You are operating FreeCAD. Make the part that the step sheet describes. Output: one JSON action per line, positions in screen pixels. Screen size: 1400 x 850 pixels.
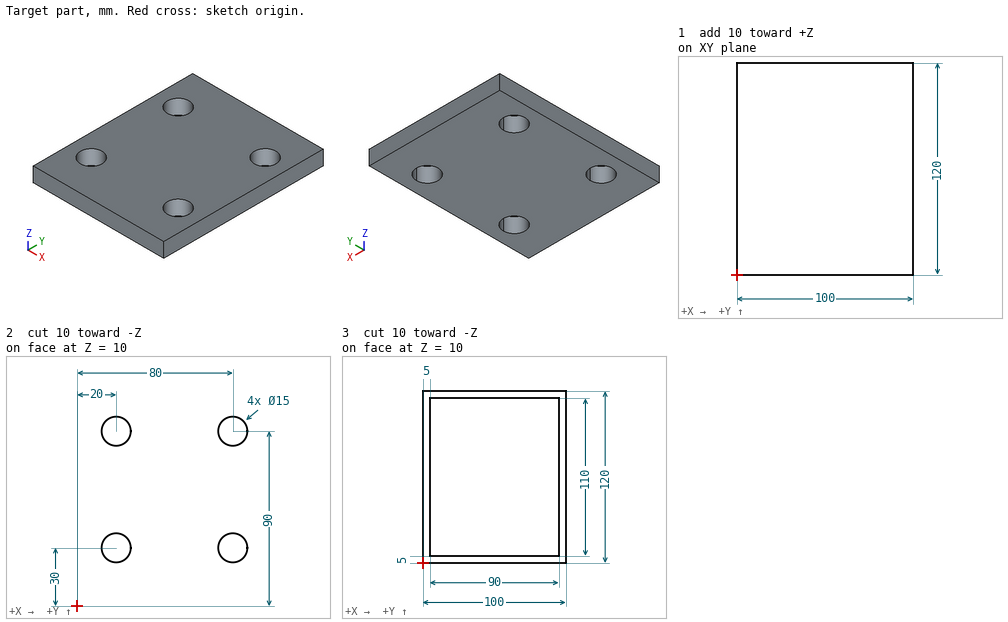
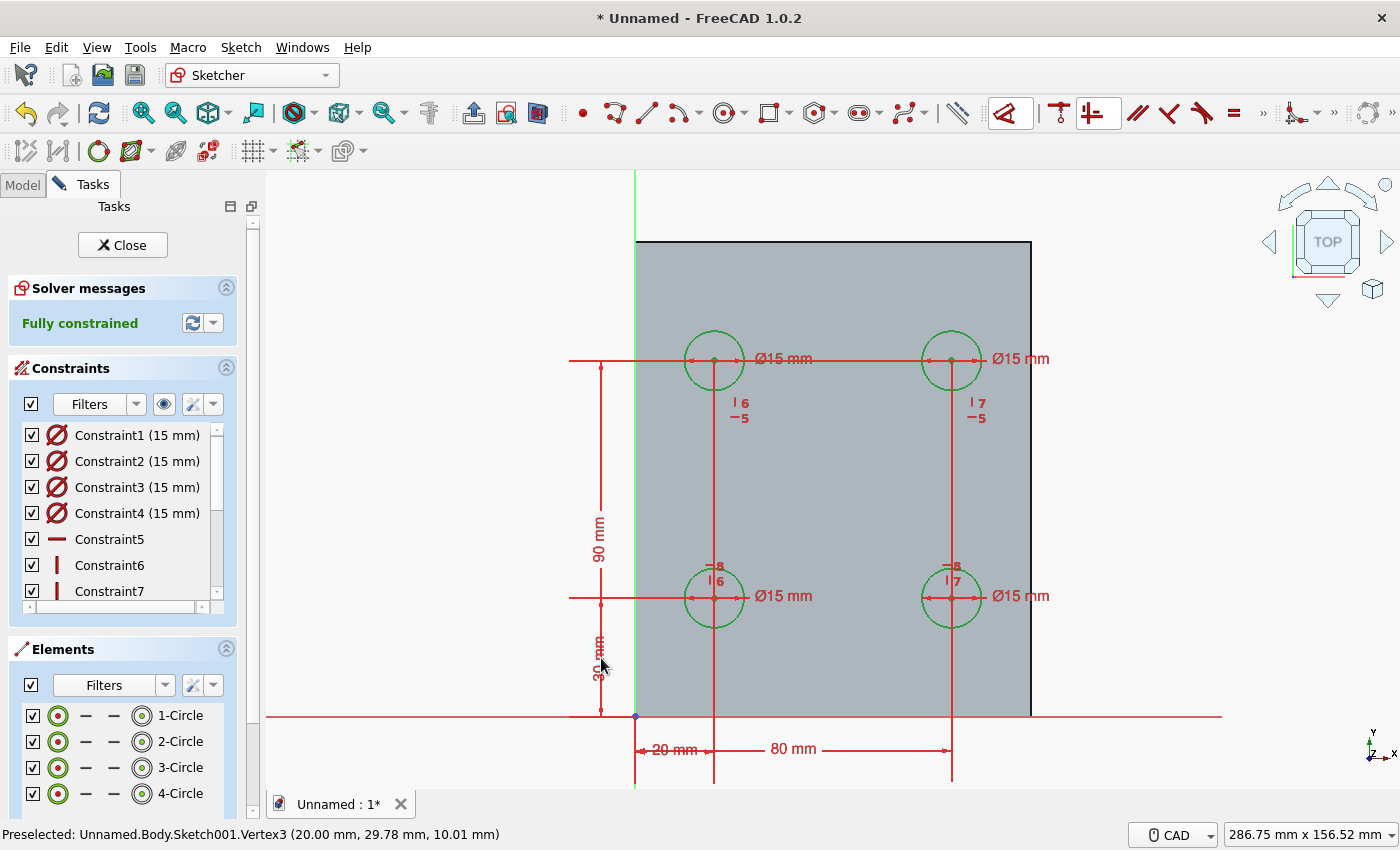
{"action": "left_click", "coordinate": [123, 245]}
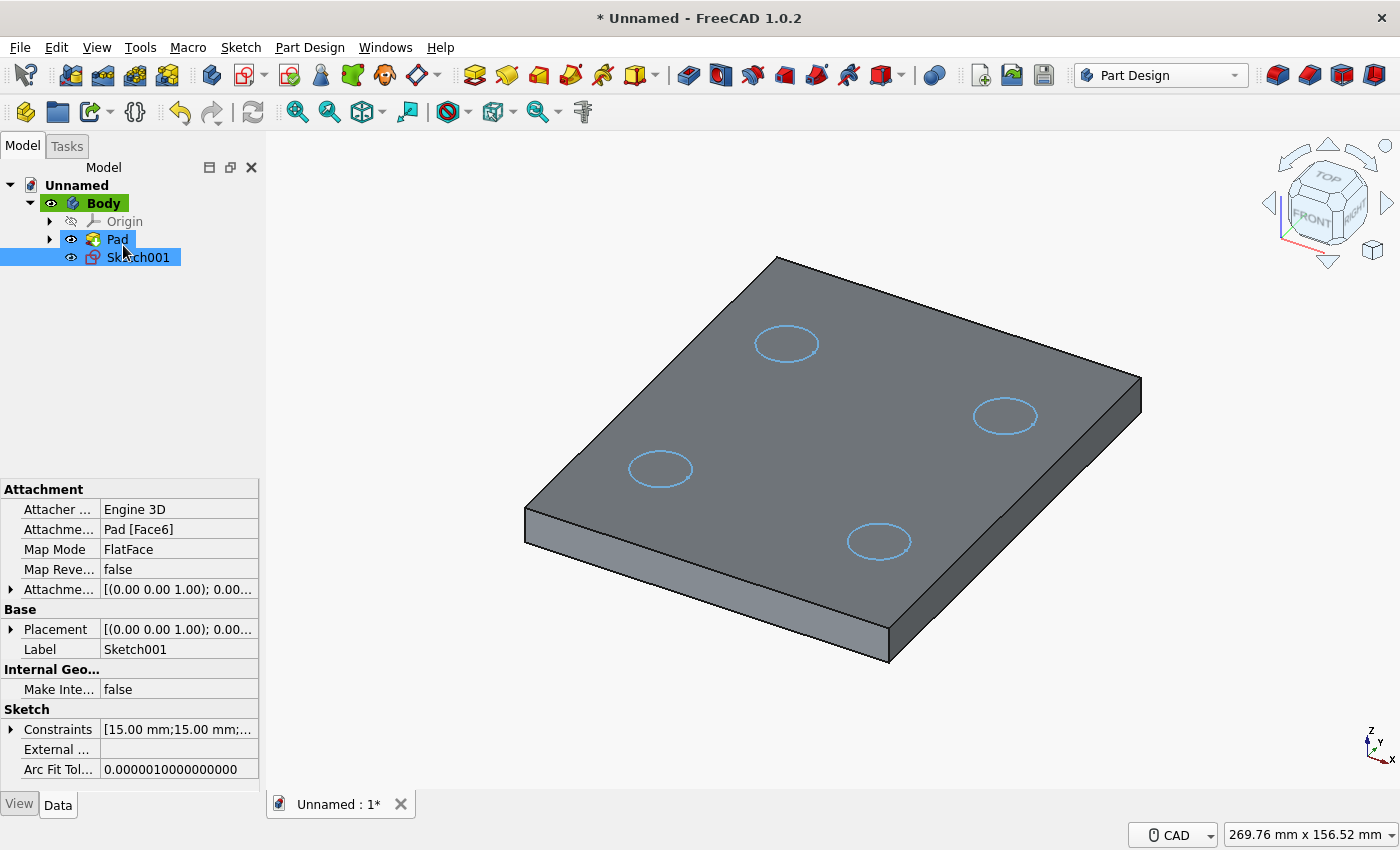
{"action": "left_click", "coordinate": [690, 76]}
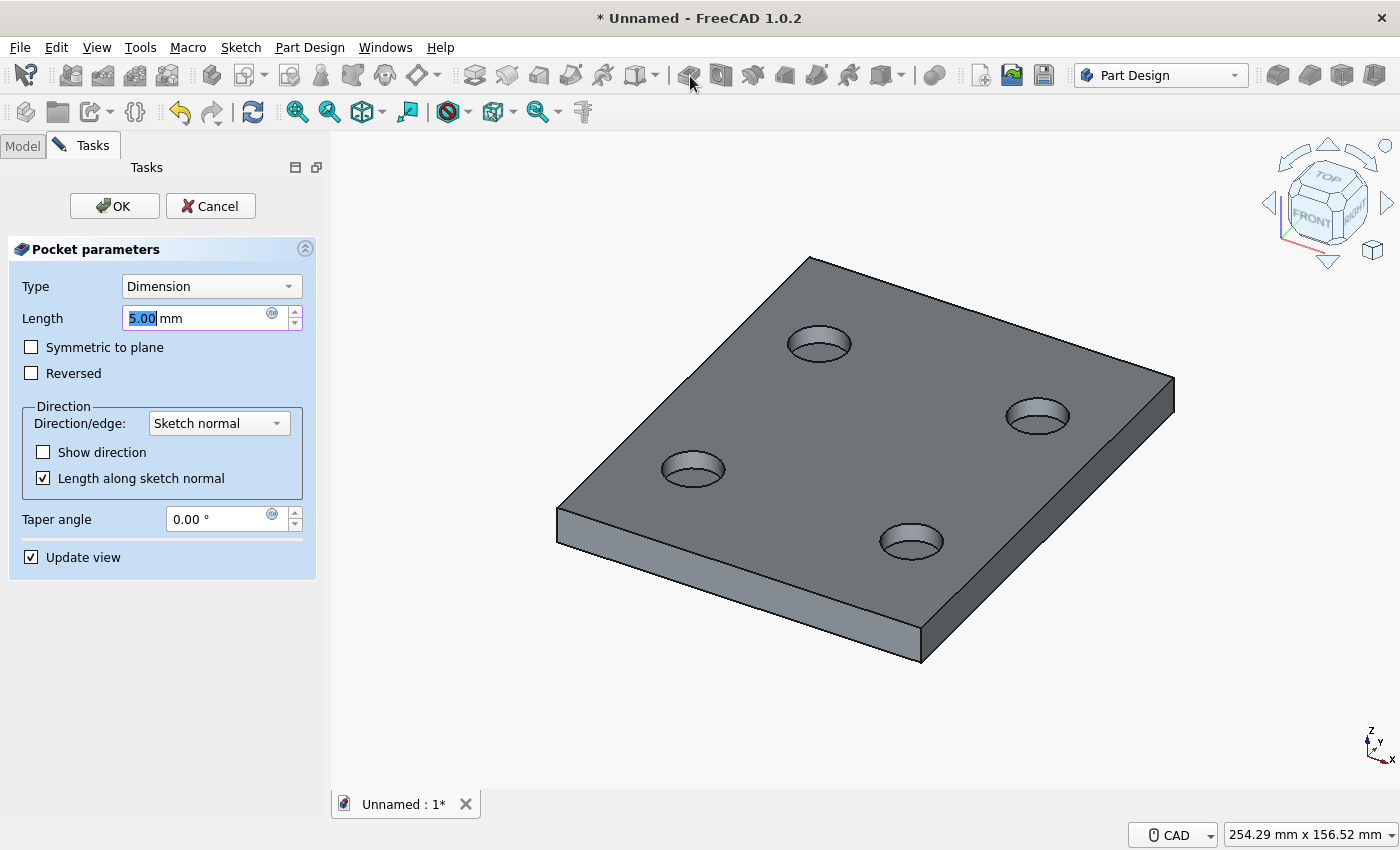
{"action": "type", "text": "10"}
{"action": "key", "text": "Tab"}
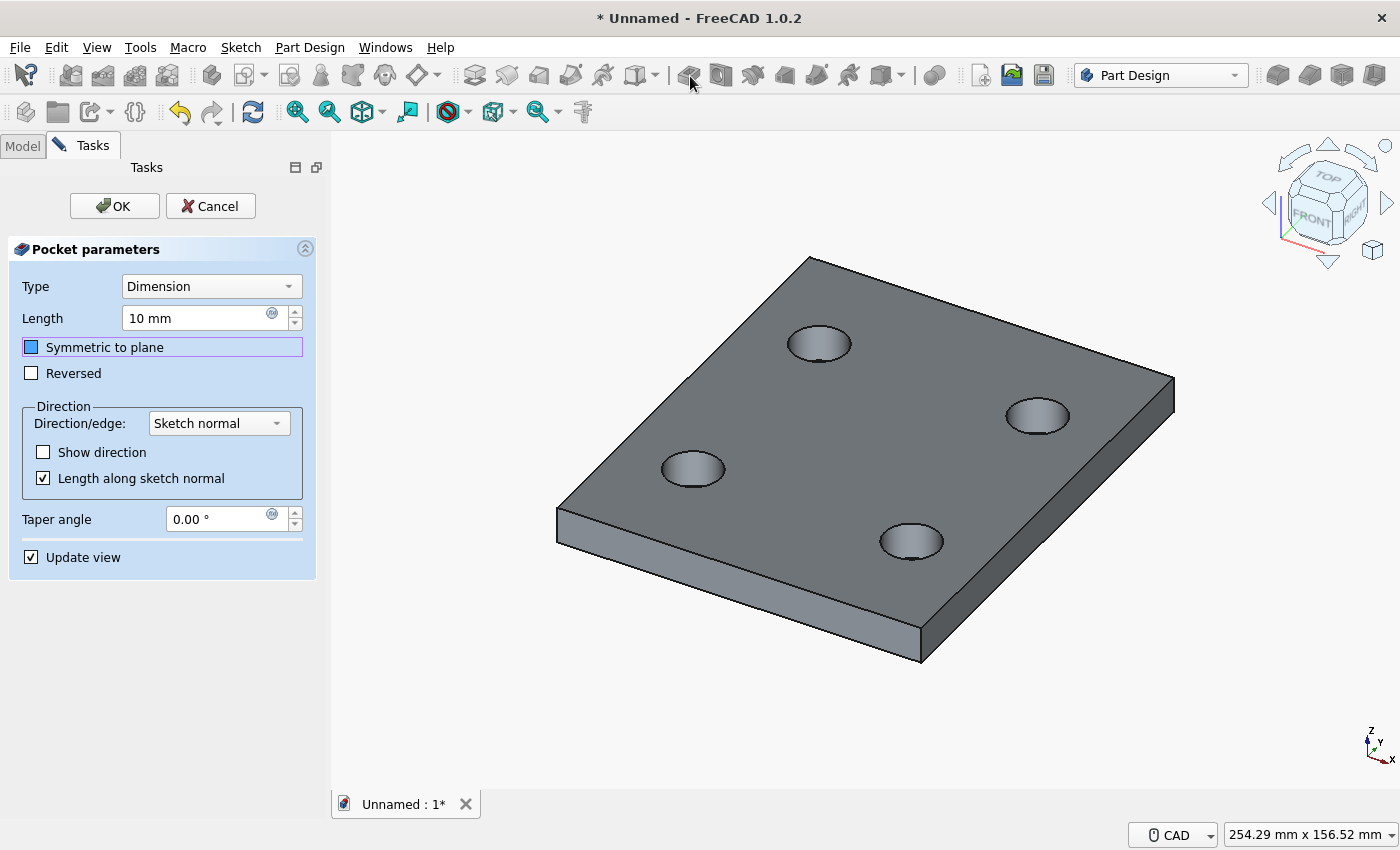
{"action": "left_click", "coordinate": [115, 206]}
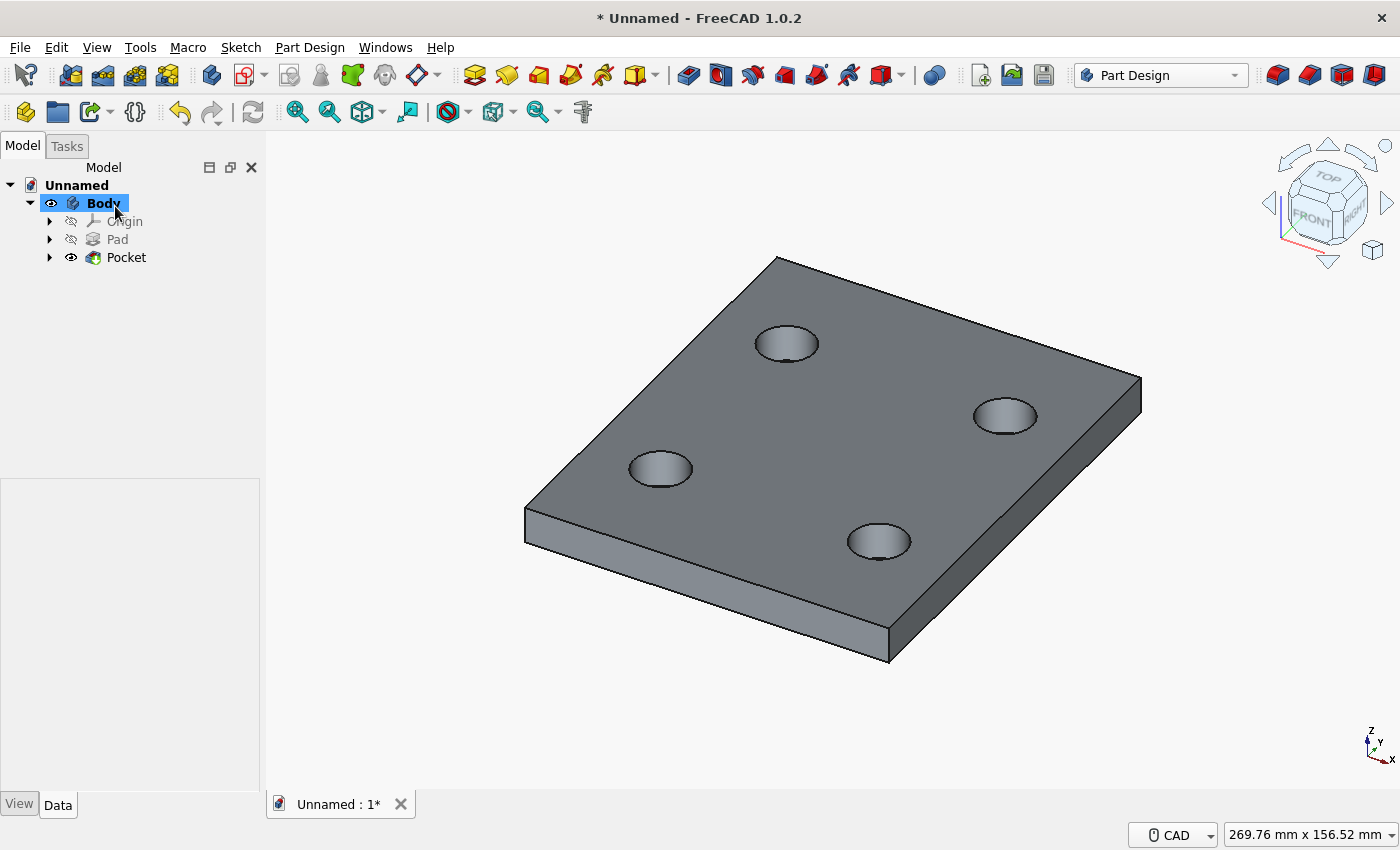
{"action": "left_click", "coordinate": [833, 442]}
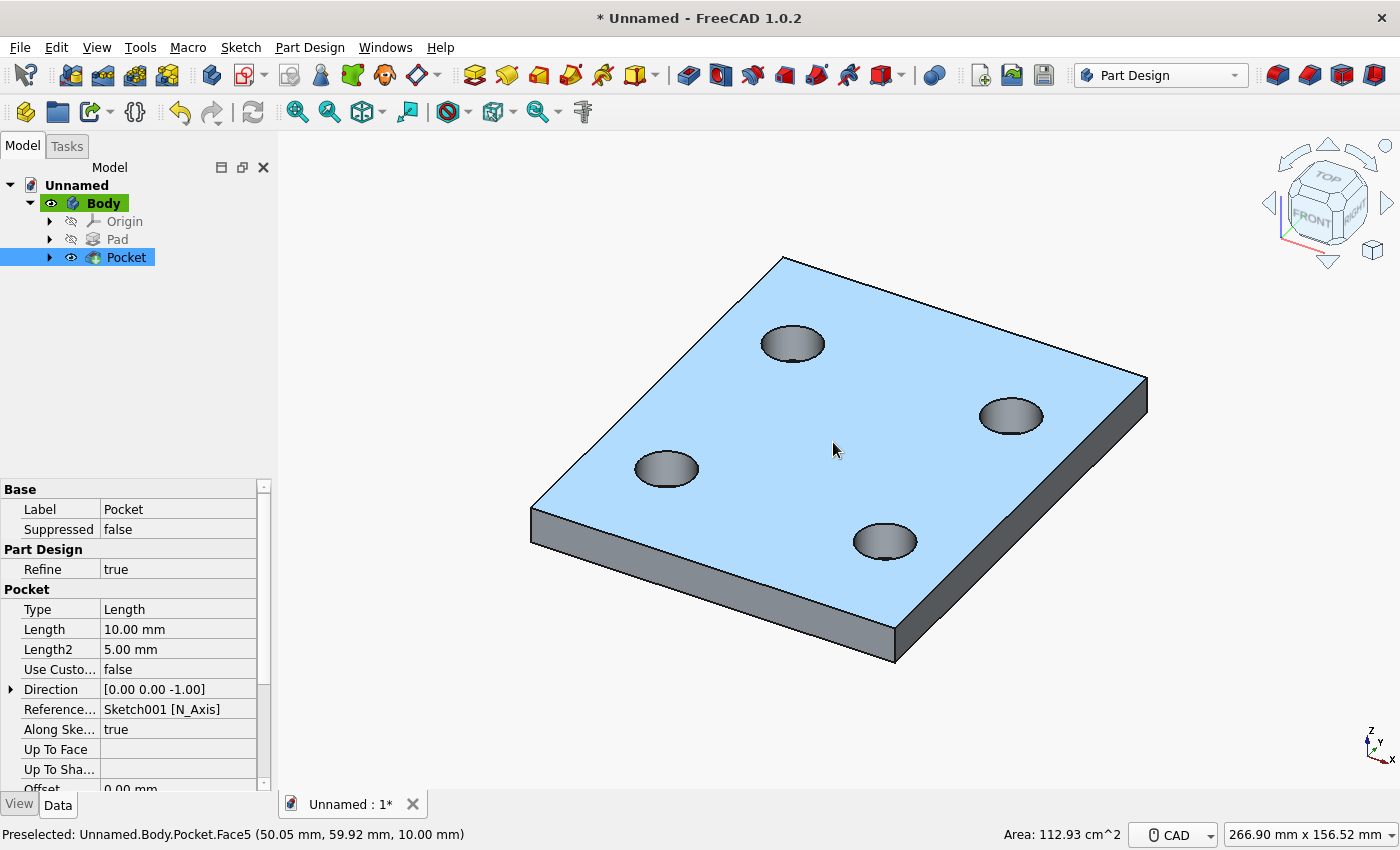
{"action": "left_click", "coordinate": [244, 76]}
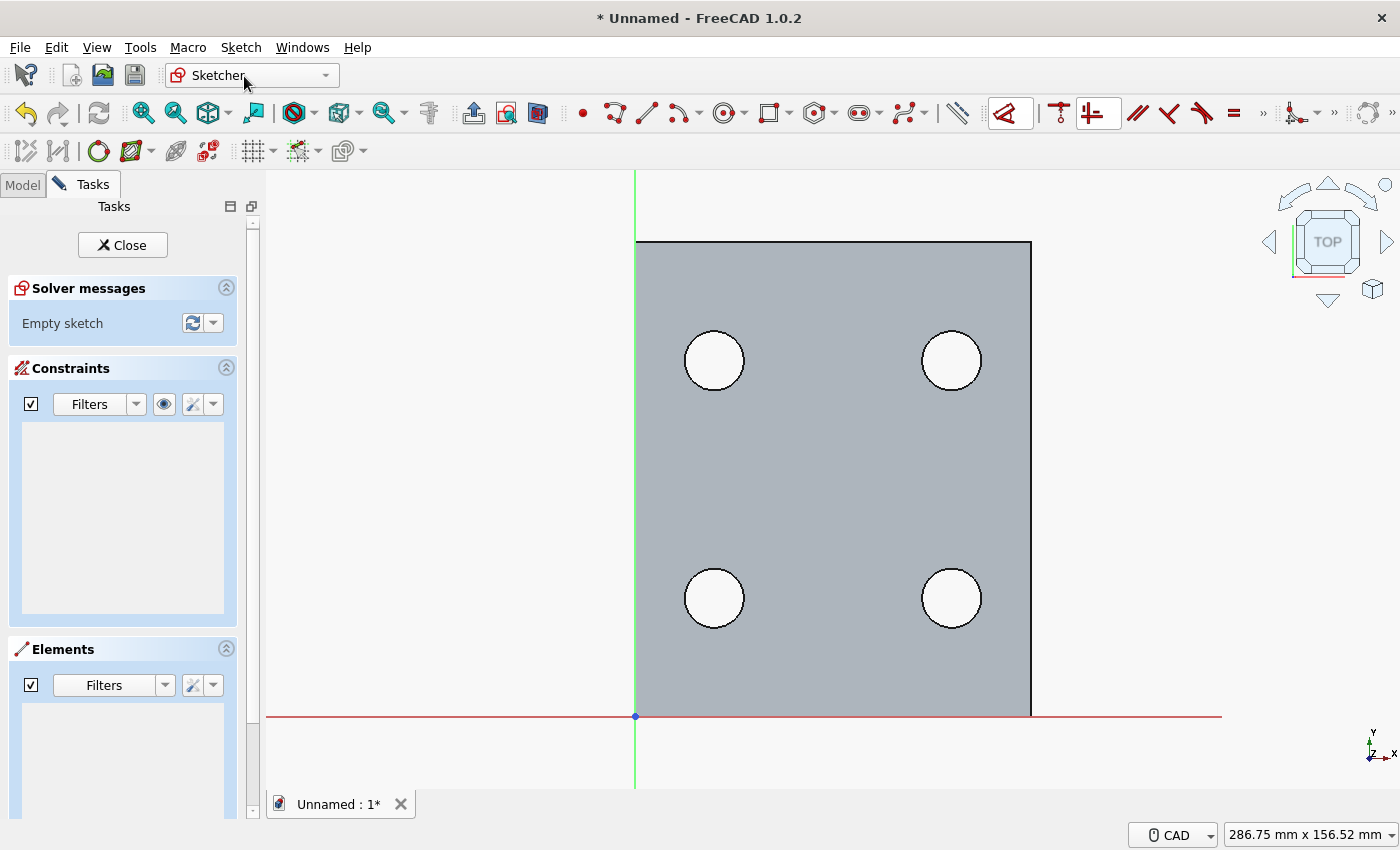
{"action": "left_click", "coordinate": [770, 114]}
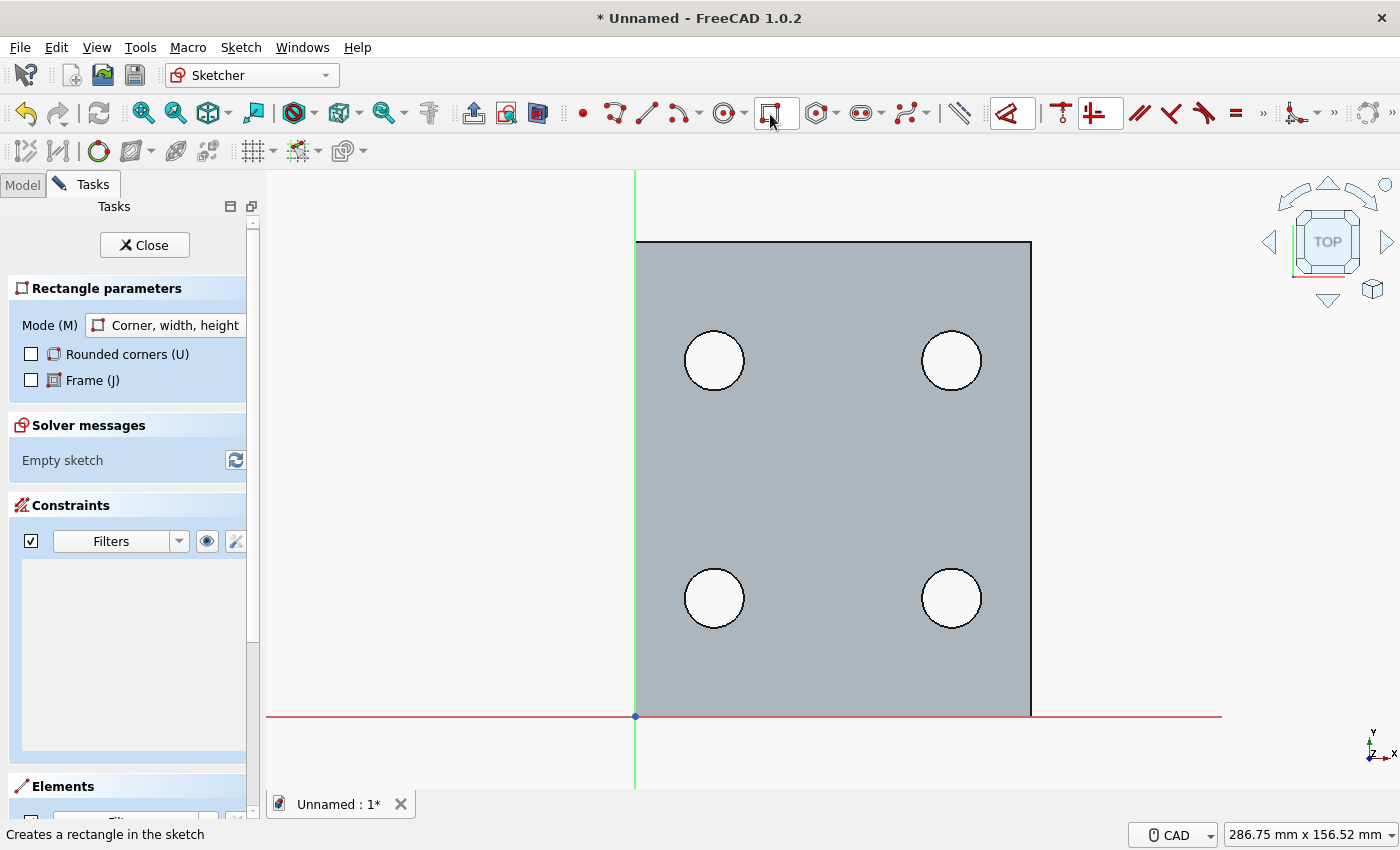
{"action": "left_click", "coordinate": [635, 717]}
{"action": "mouse_move", "coordinate": [1031, 242]}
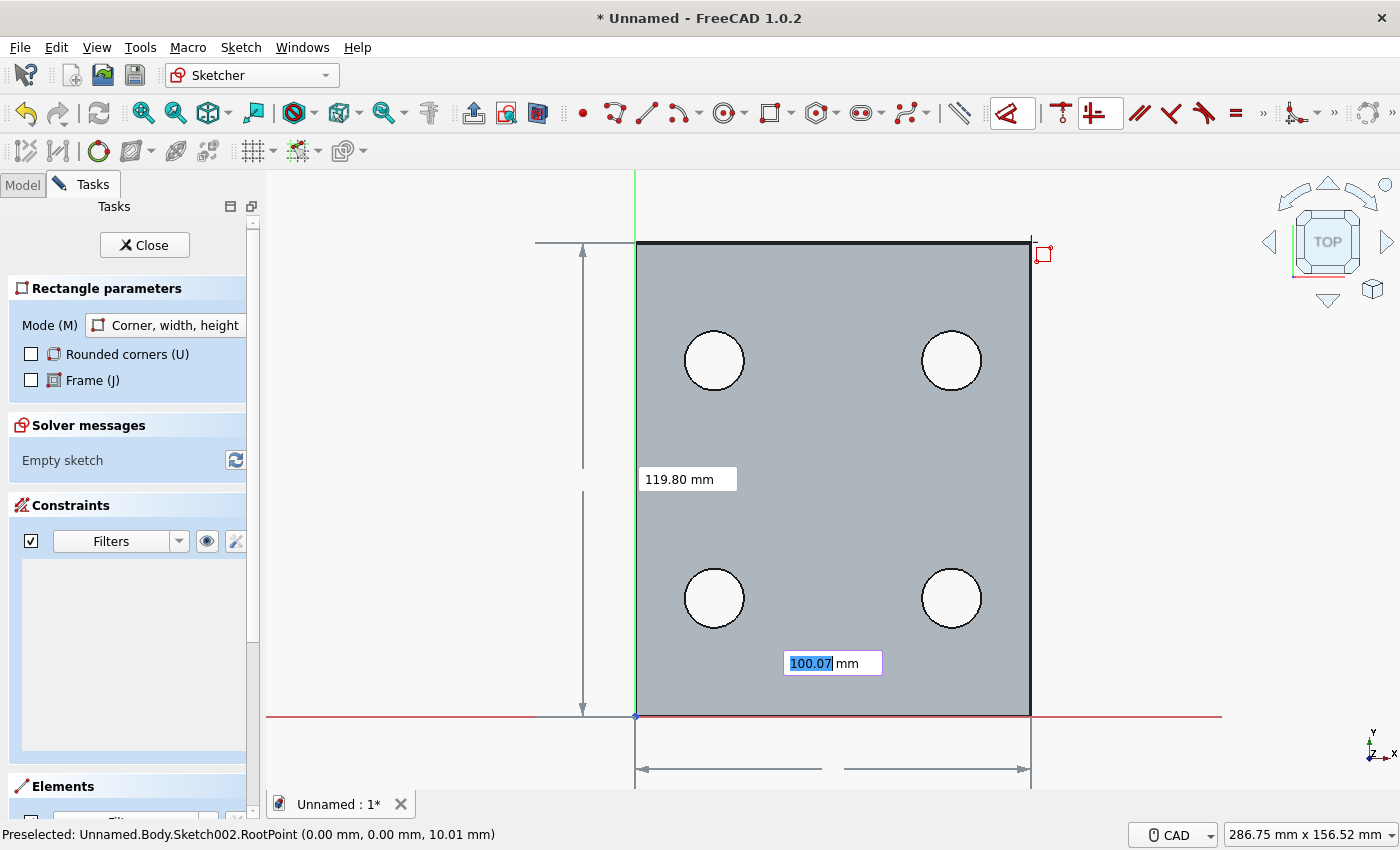
{"action": "type", "text": "100"}
{"action": "key", "text": "Tab"}
{"action": "type", "text": "120"}
{"action": "key", "text": "Return"}